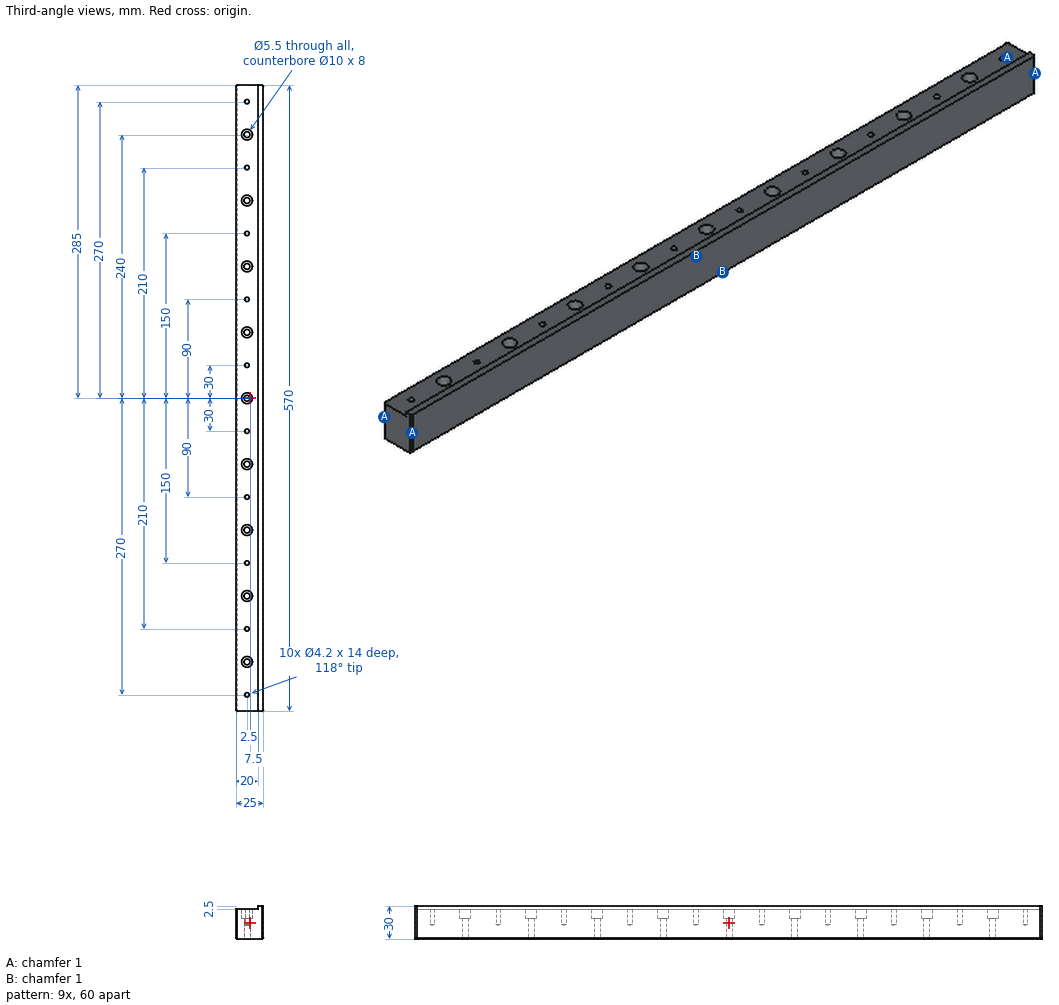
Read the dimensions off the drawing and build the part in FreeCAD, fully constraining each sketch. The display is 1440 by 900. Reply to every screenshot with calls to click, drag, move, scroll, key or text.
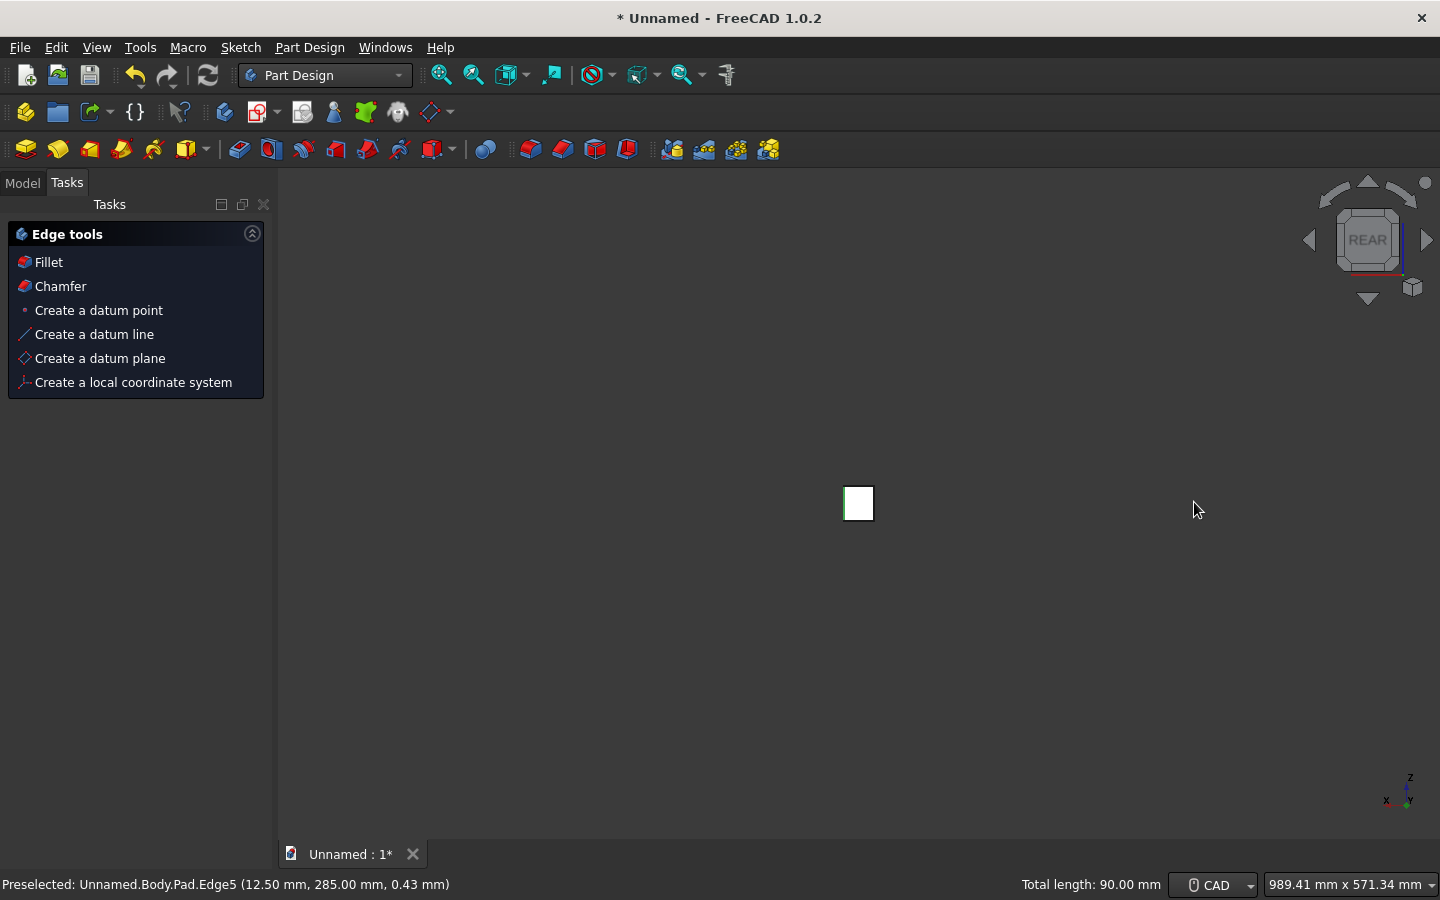
click(874, 503, ctrl)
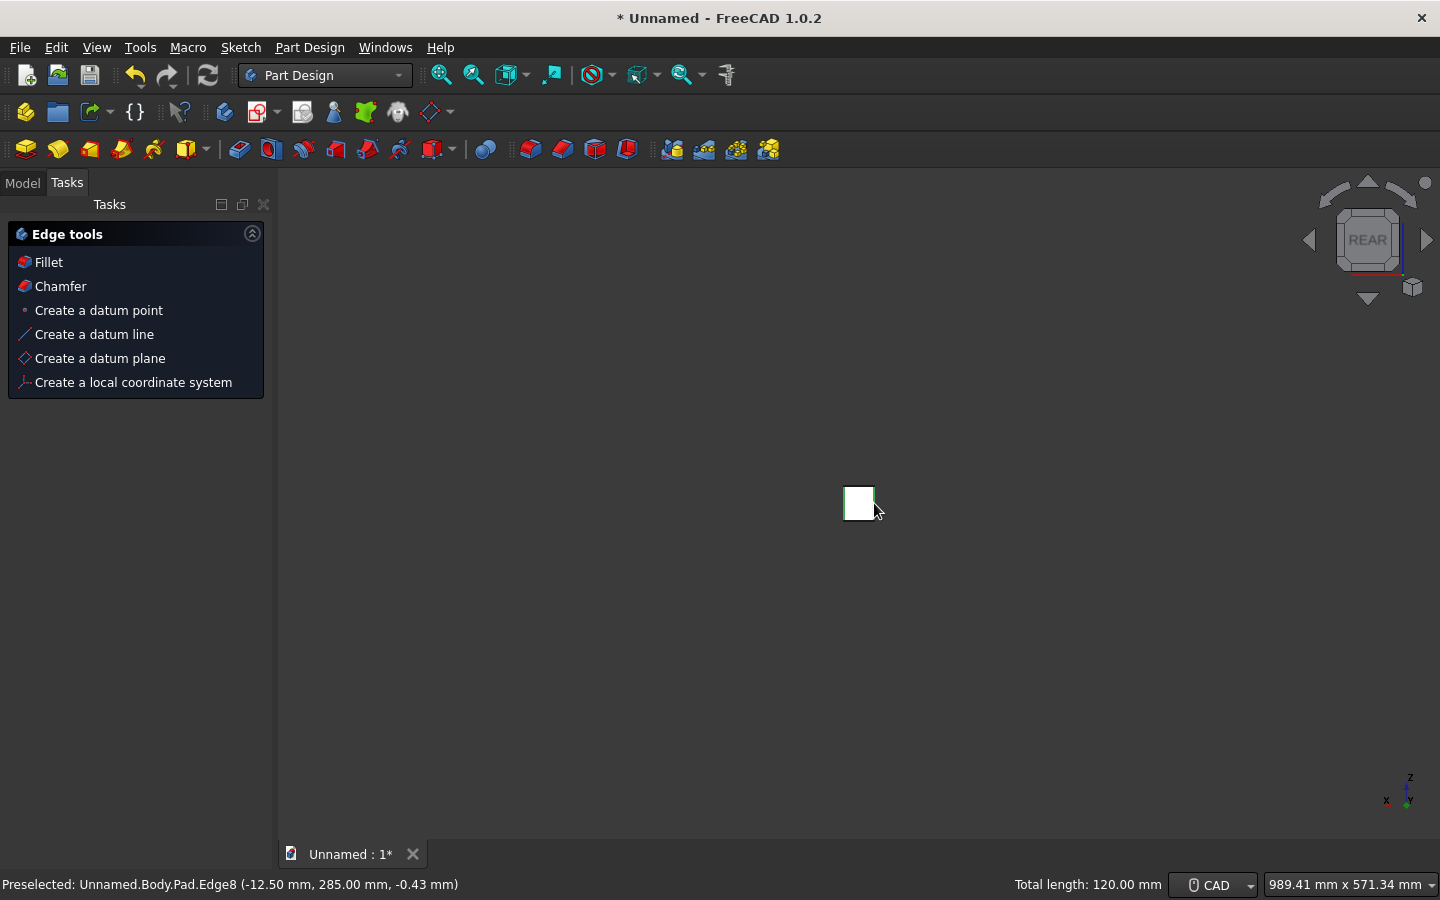
click(564, 150)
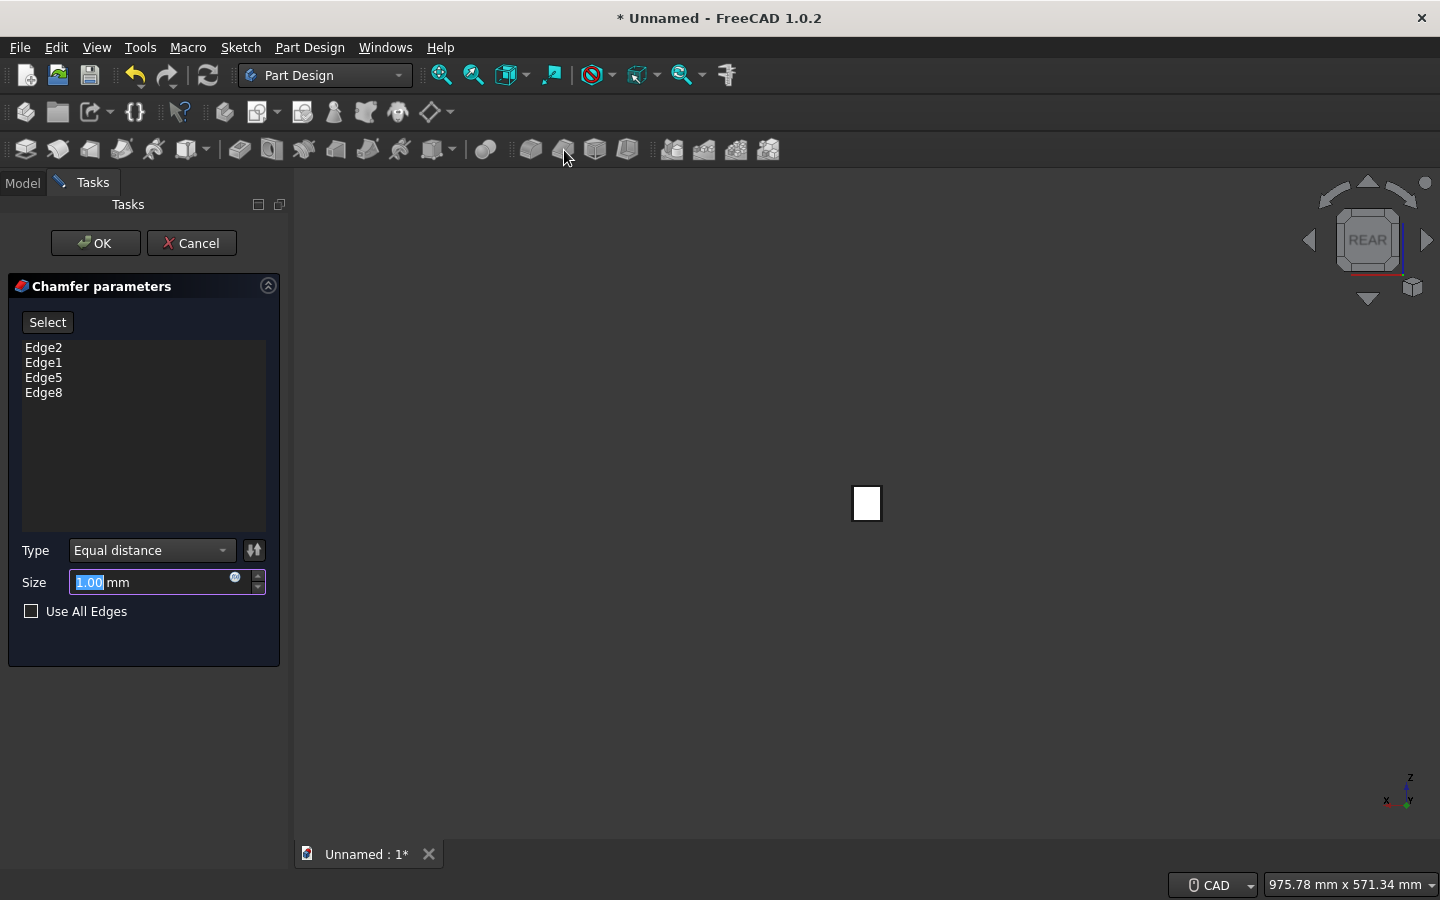
text(1)
key(Tab)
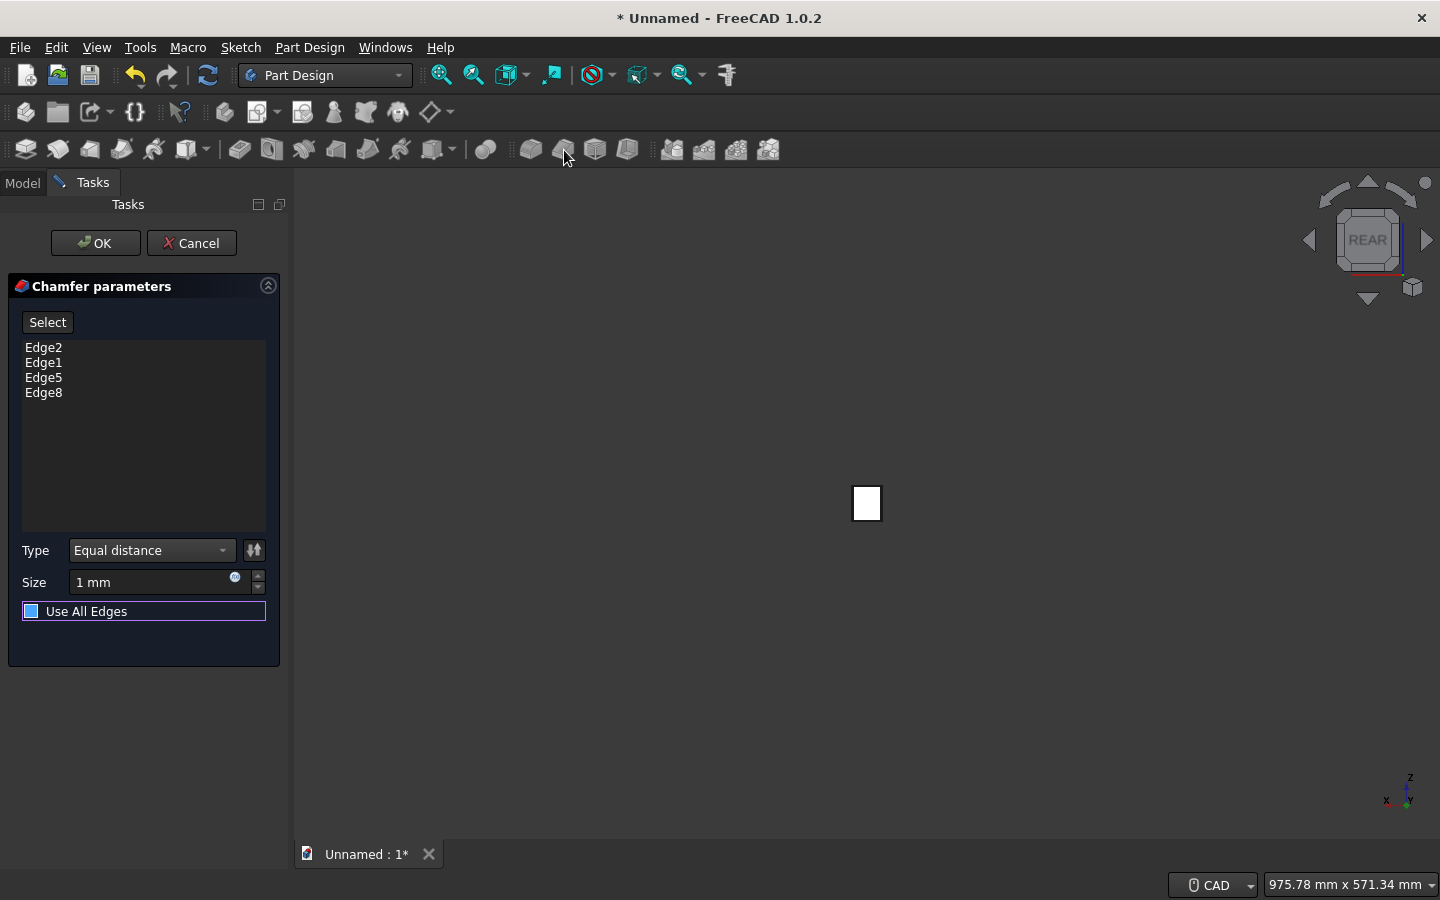
click(96, 243)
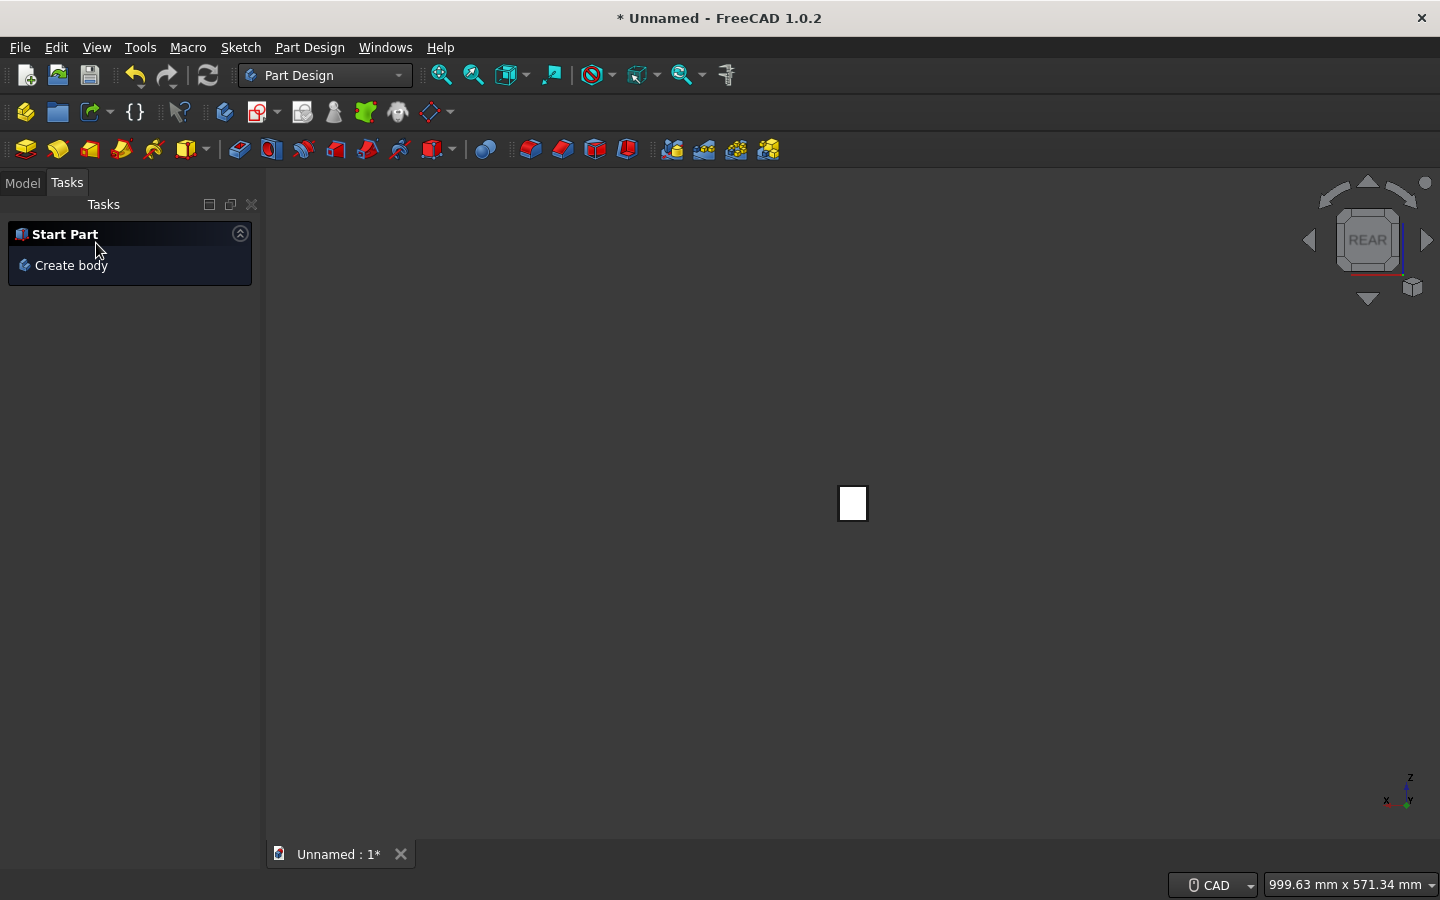
key(v)
key(f)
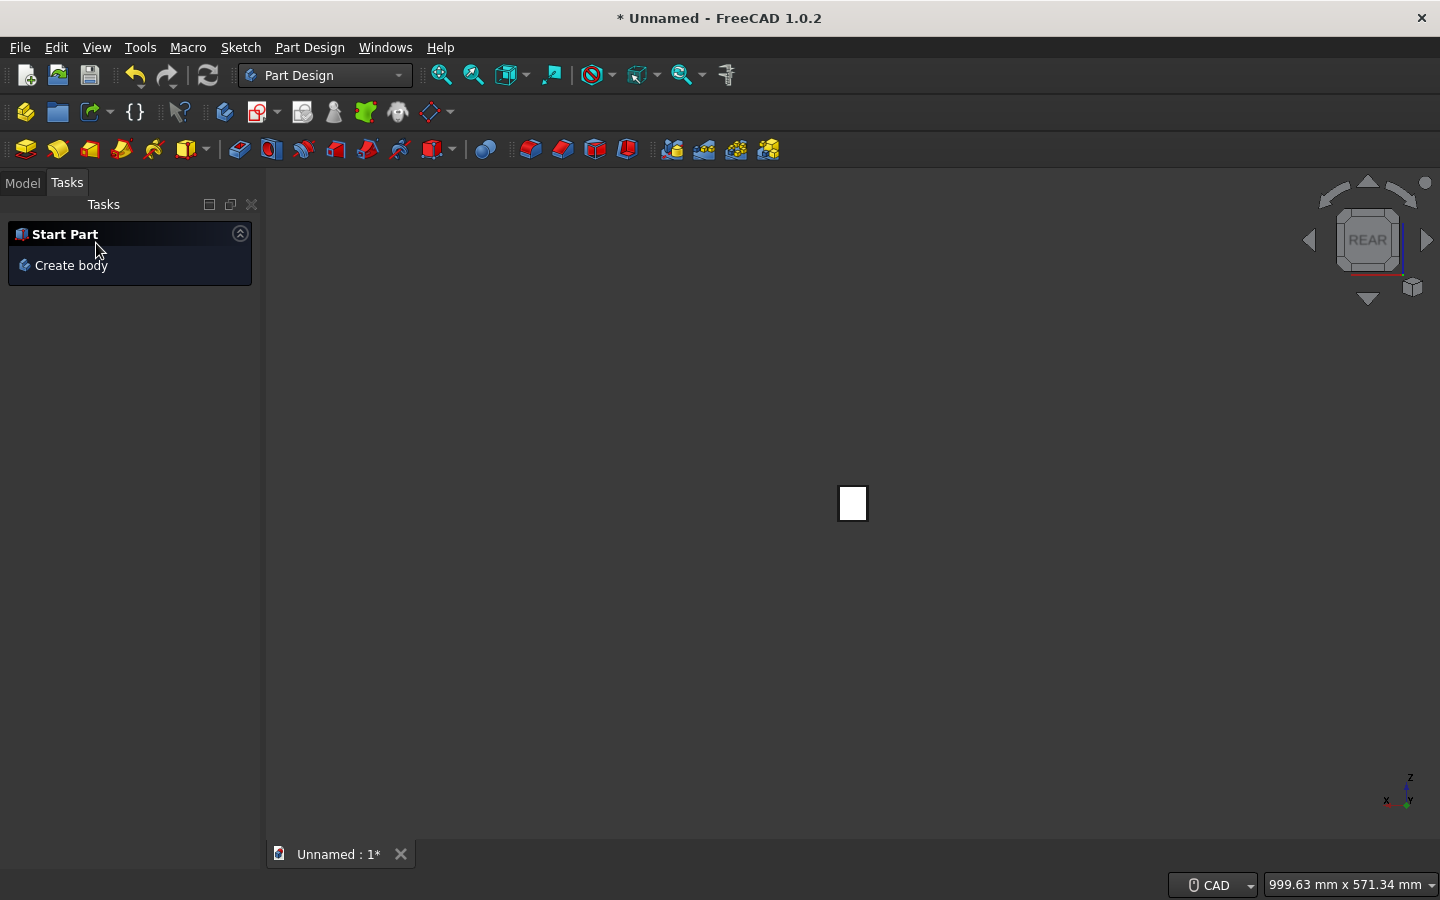
key(0)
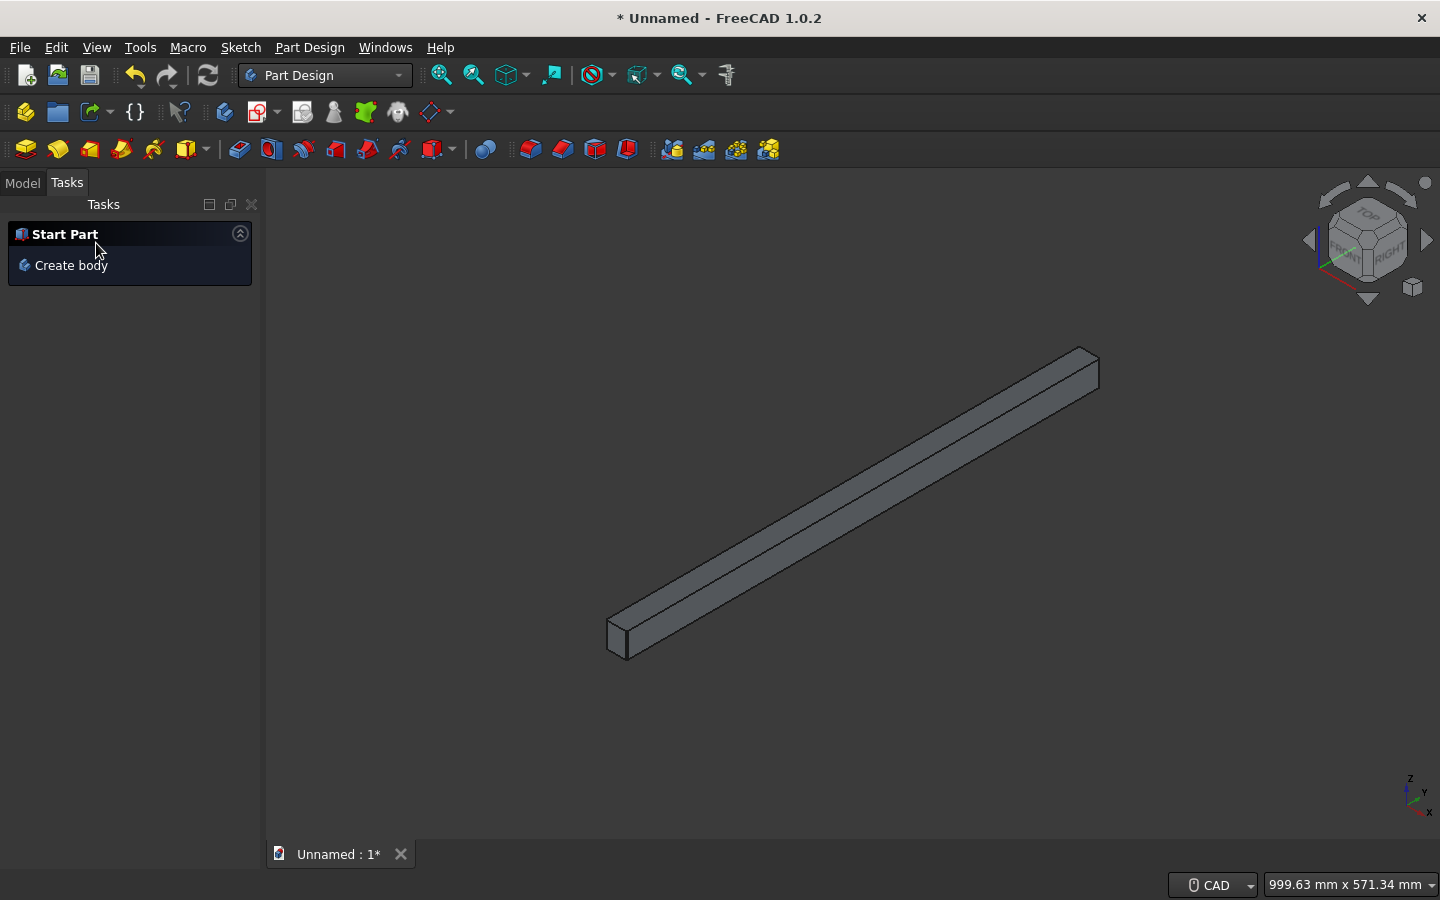
click(1056, 371)